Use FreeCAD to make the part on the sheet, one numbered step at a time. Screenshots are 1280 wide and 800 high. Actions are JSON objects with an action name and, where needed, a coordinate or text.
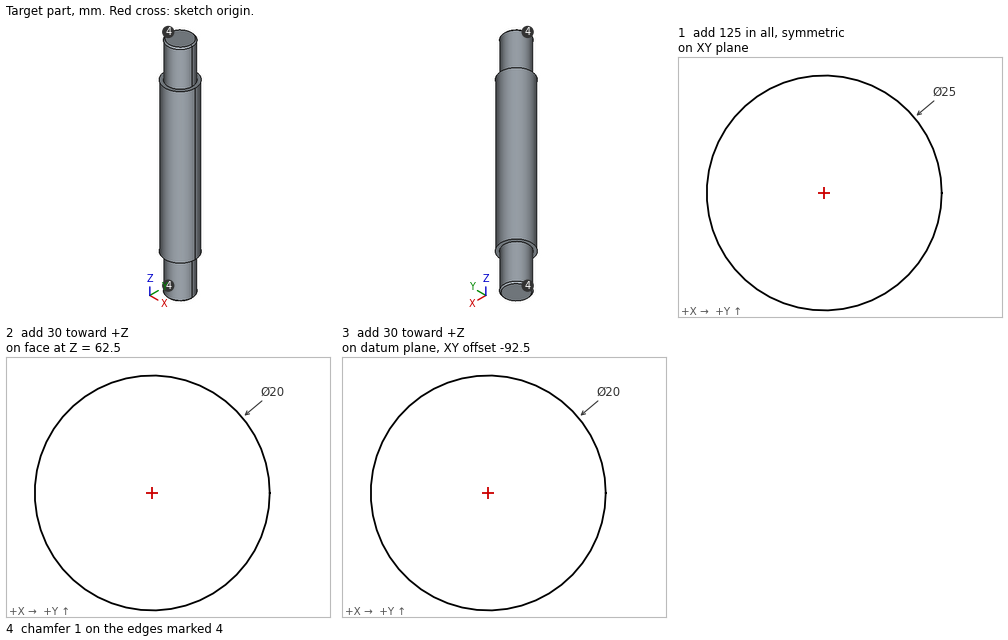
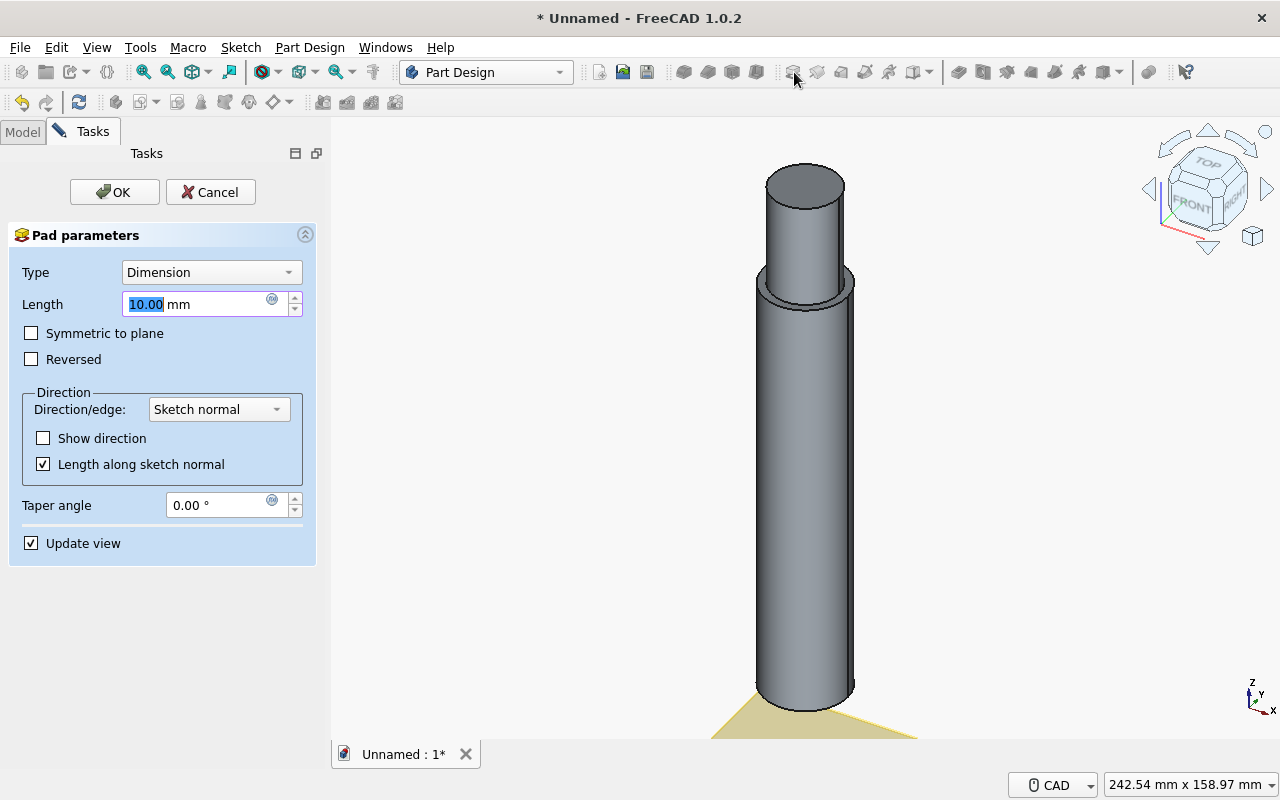
{"action": "type", "text": "30"}
{"action": "key", "text": "Tab"}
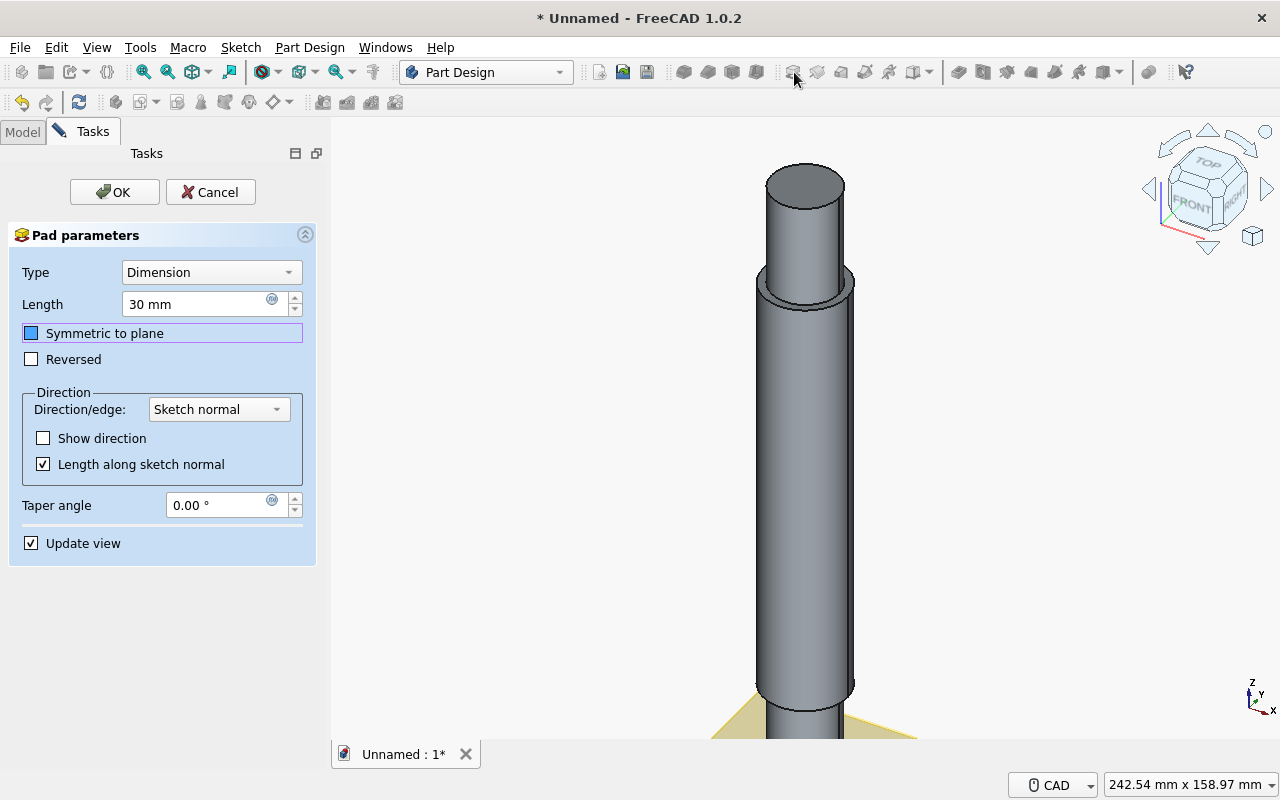
{"action": "left_click", "coordinate": [115, 192]}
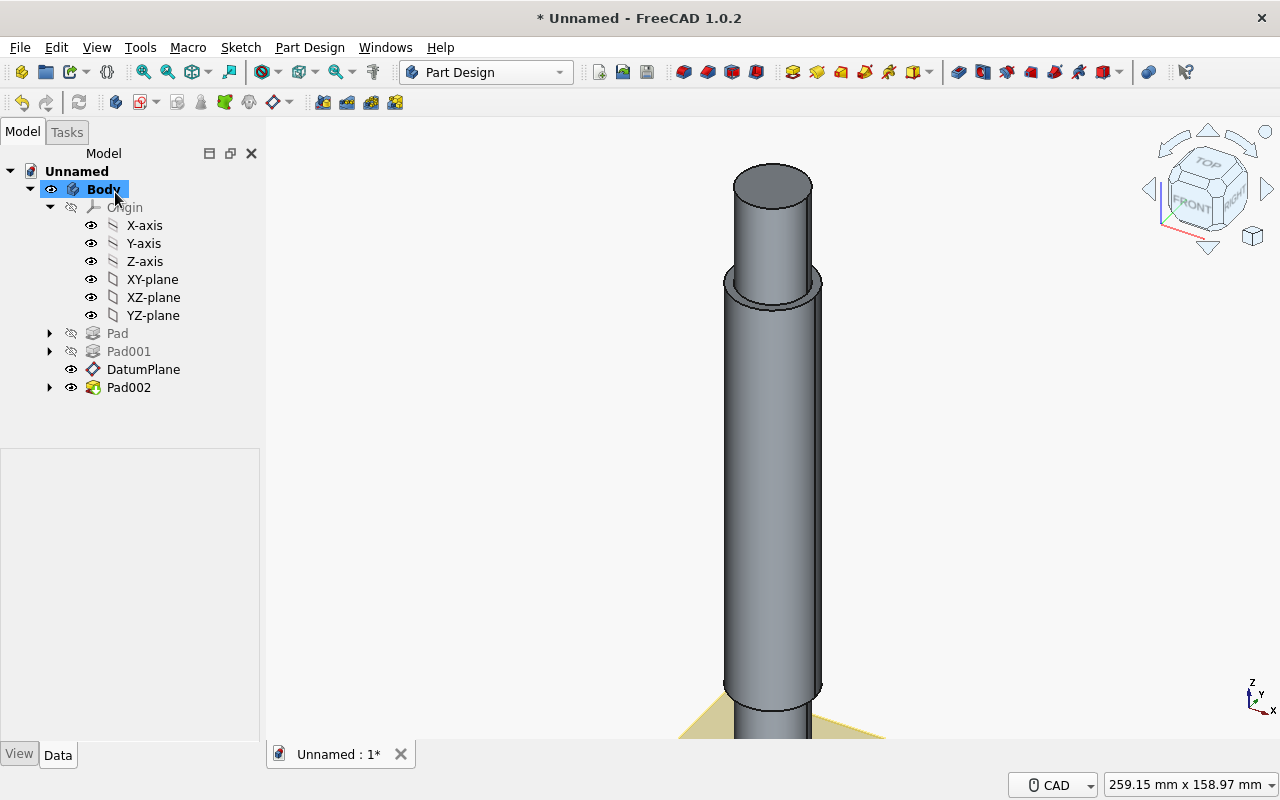
{"action": "left_click", "coordinate": [116, 369]}
{"action": "key", "text": "space"}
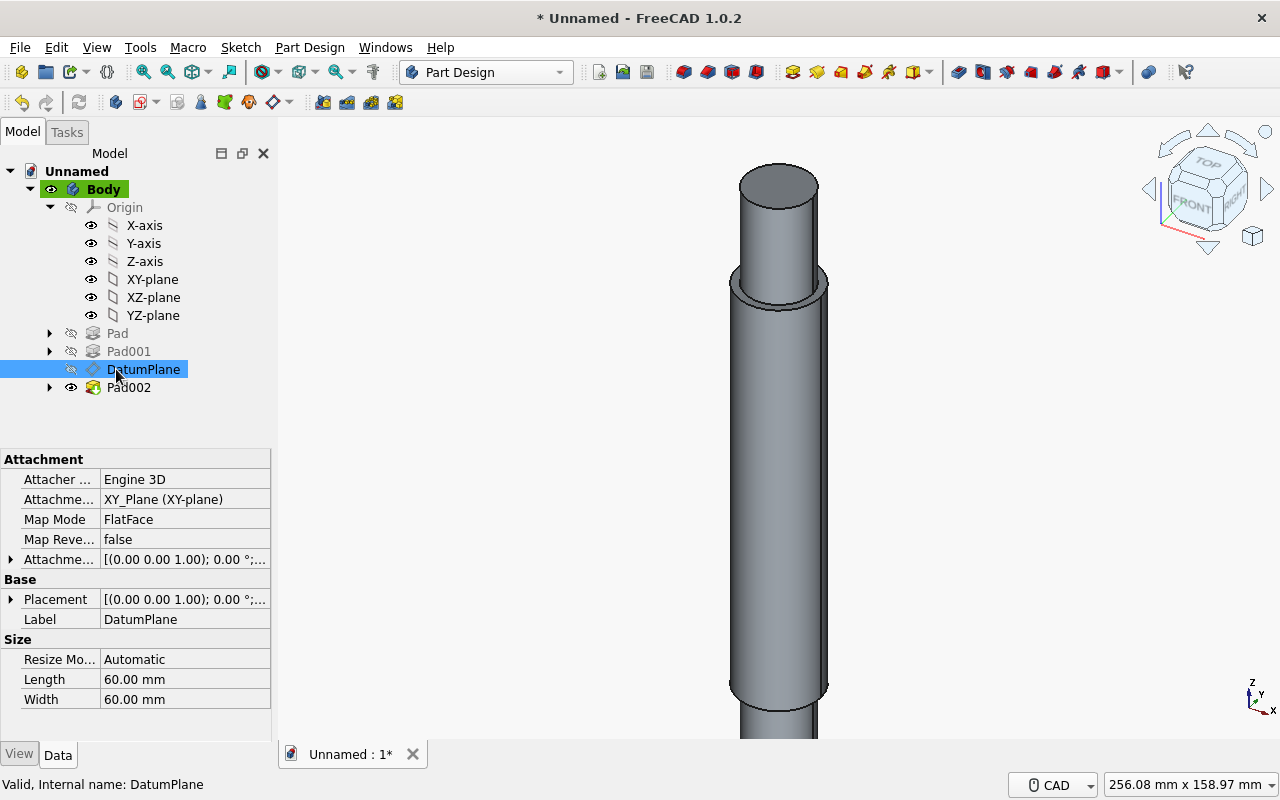
{"action": "left_click", "coordinate": [144, 72]}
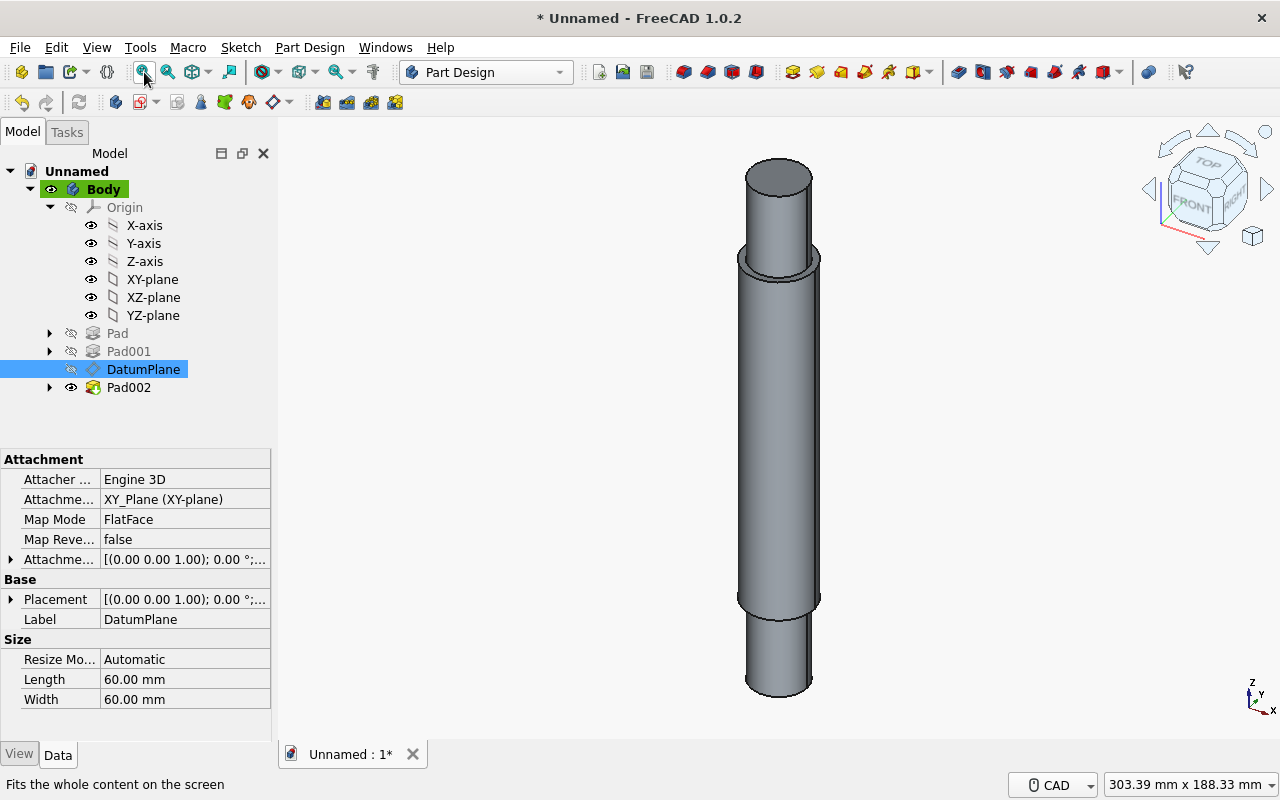
{"action": "left_click", "coordinate": [746, 179]}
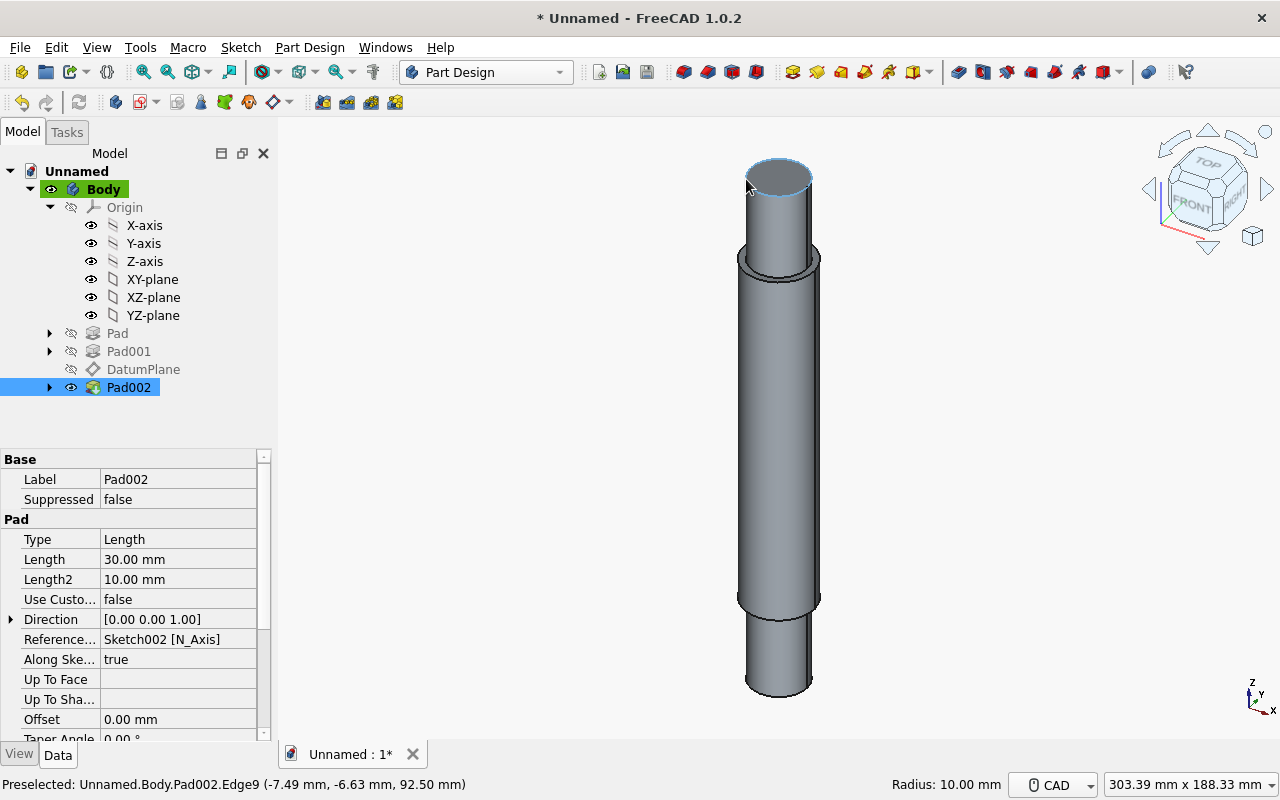
{"action": "key", "text": "0"}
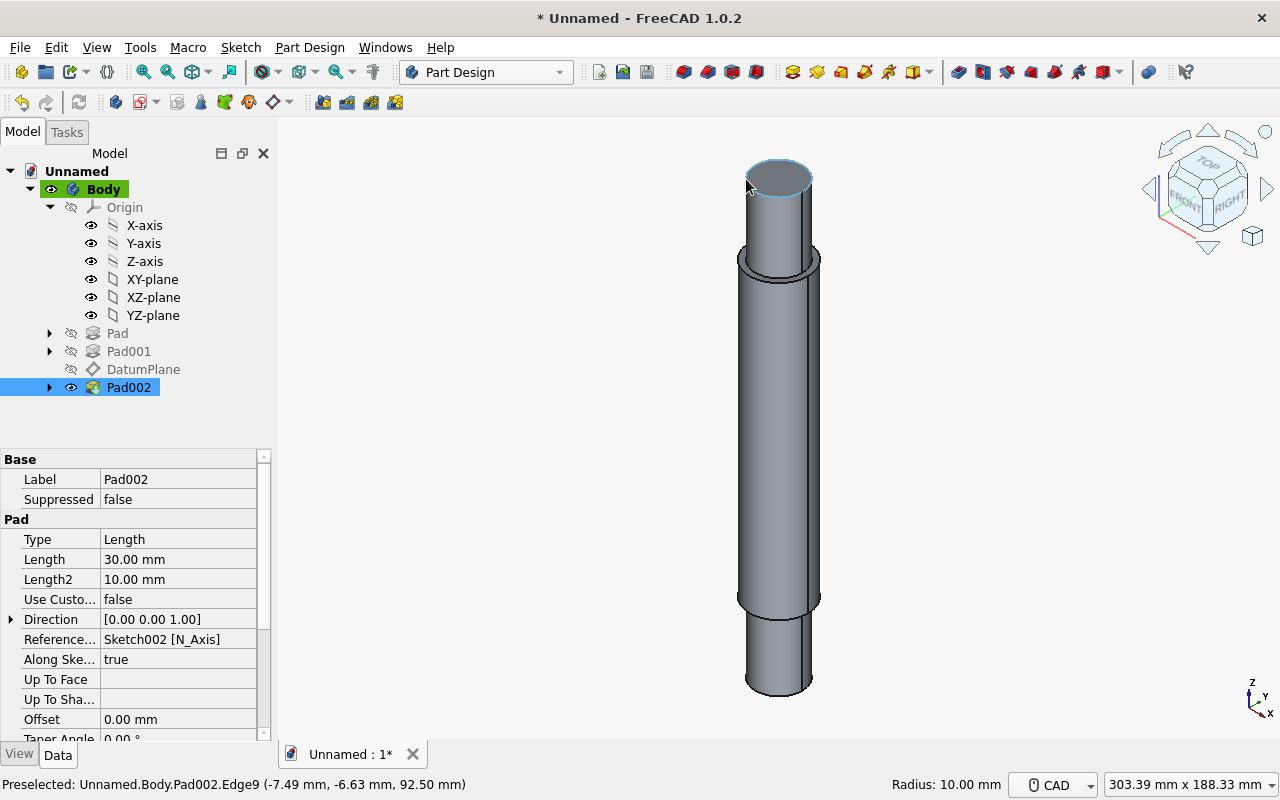
{"action": "key", "text": "2"}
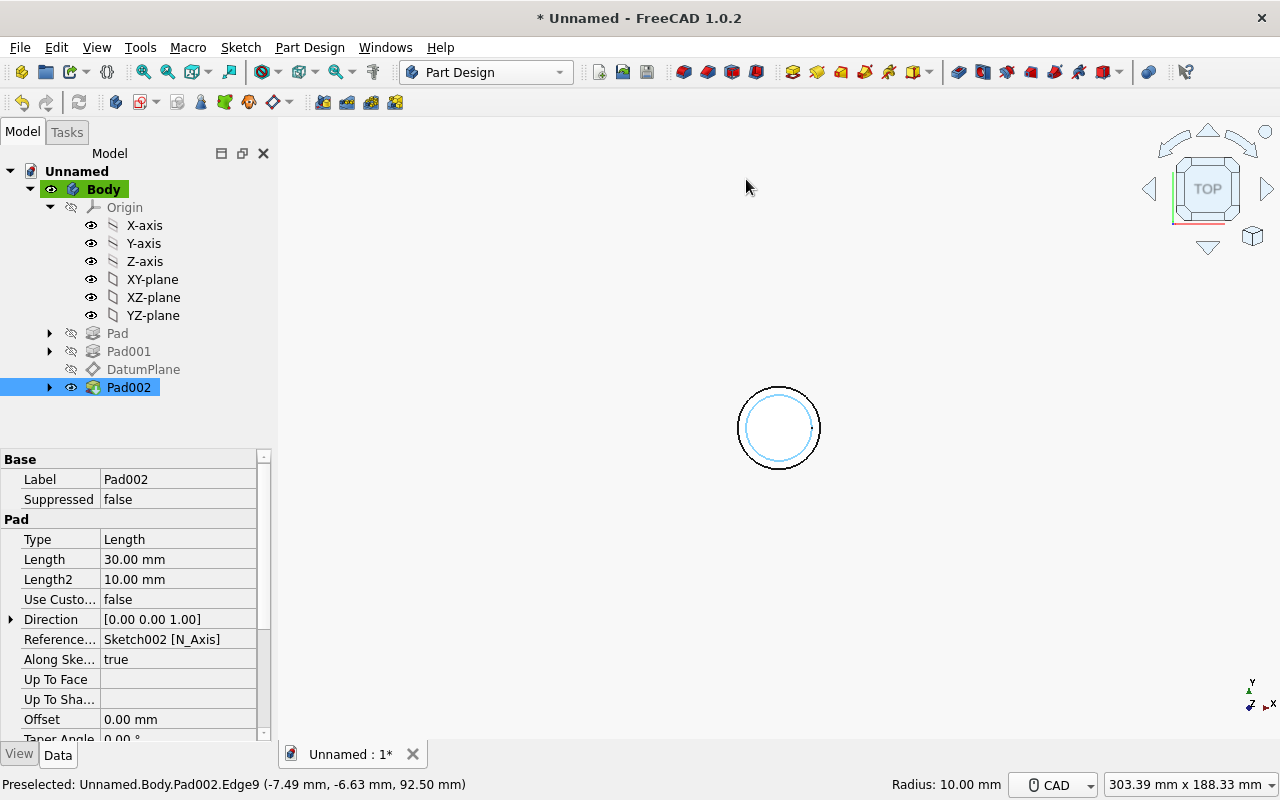
{"action": "left_click", "coordinate": [144, 72]}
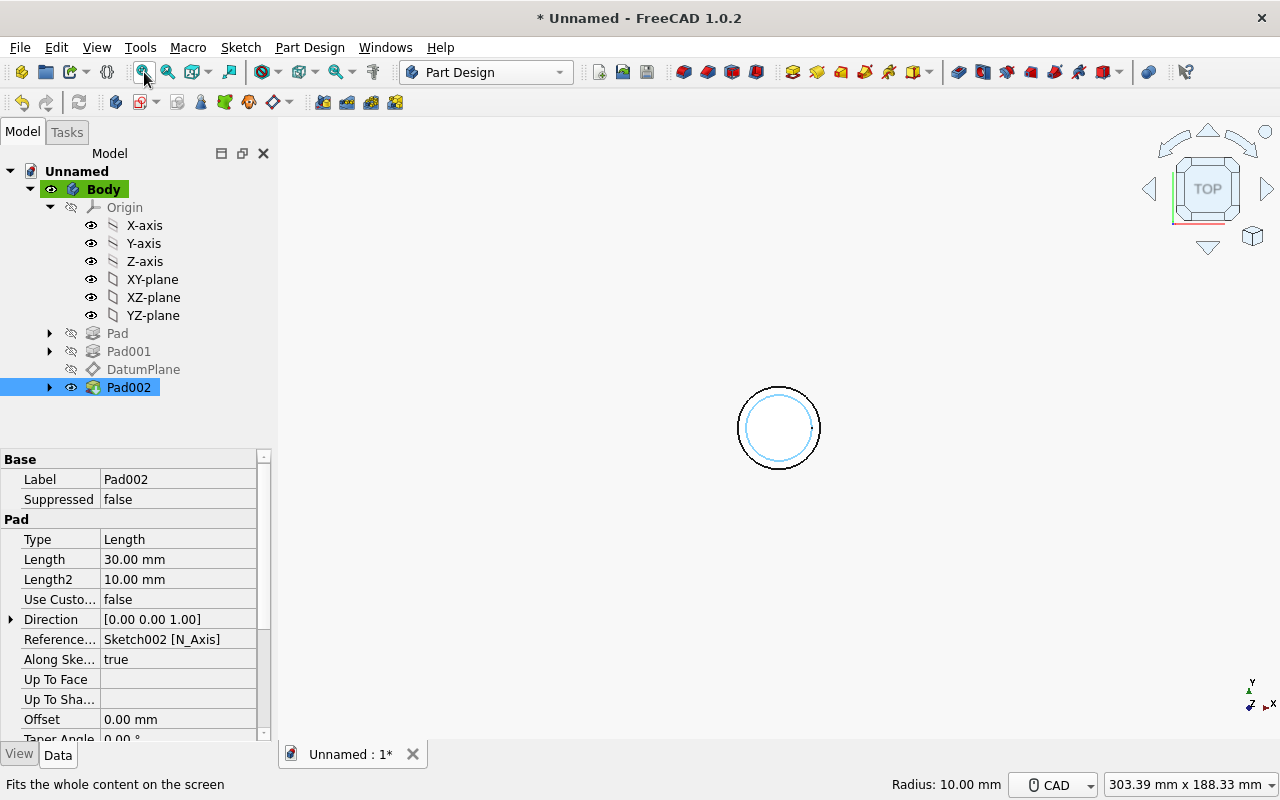
{"action": "key", "text": "1"}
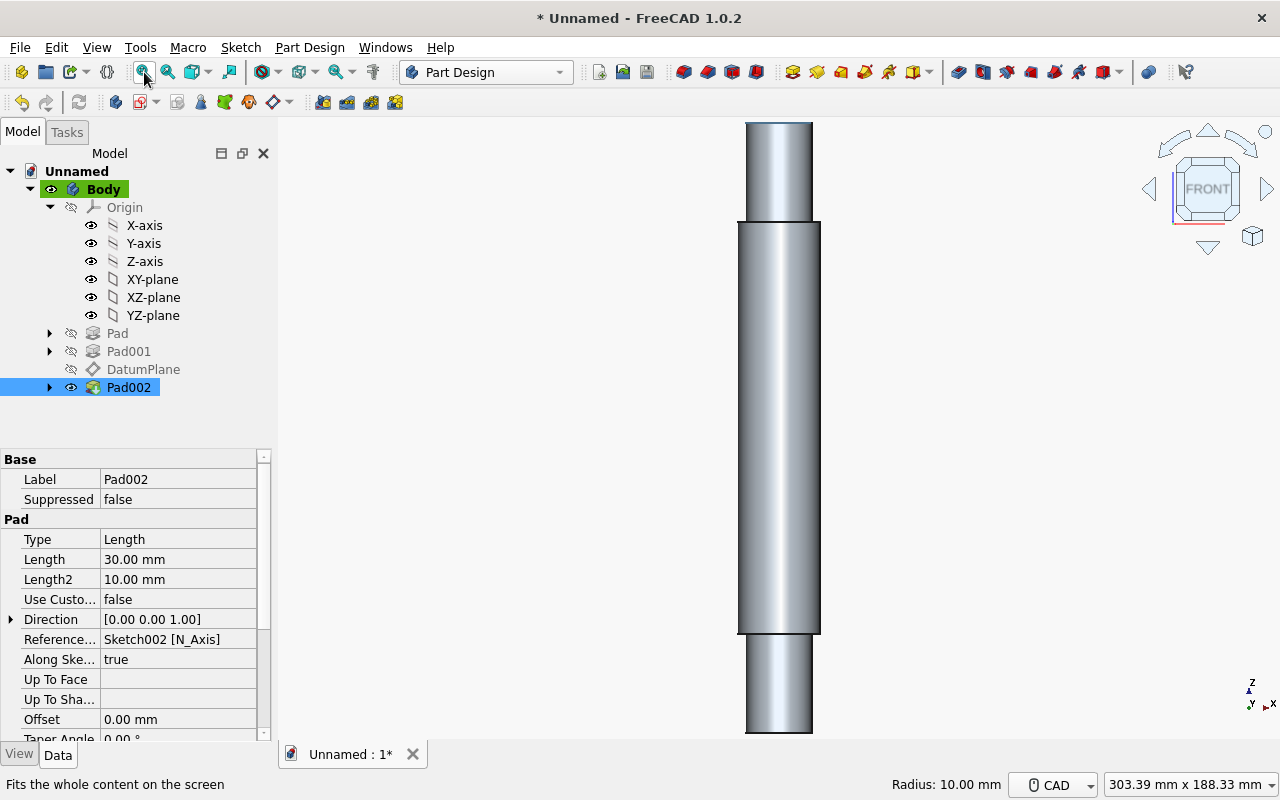
{"action": "key", "text": "3"}